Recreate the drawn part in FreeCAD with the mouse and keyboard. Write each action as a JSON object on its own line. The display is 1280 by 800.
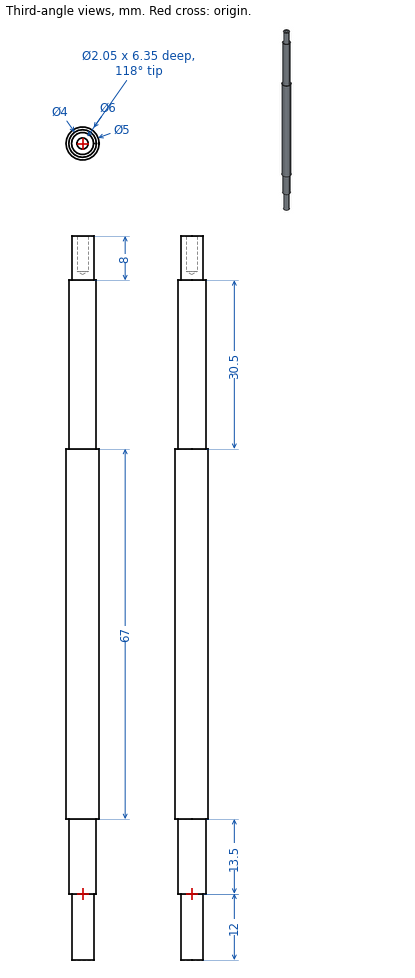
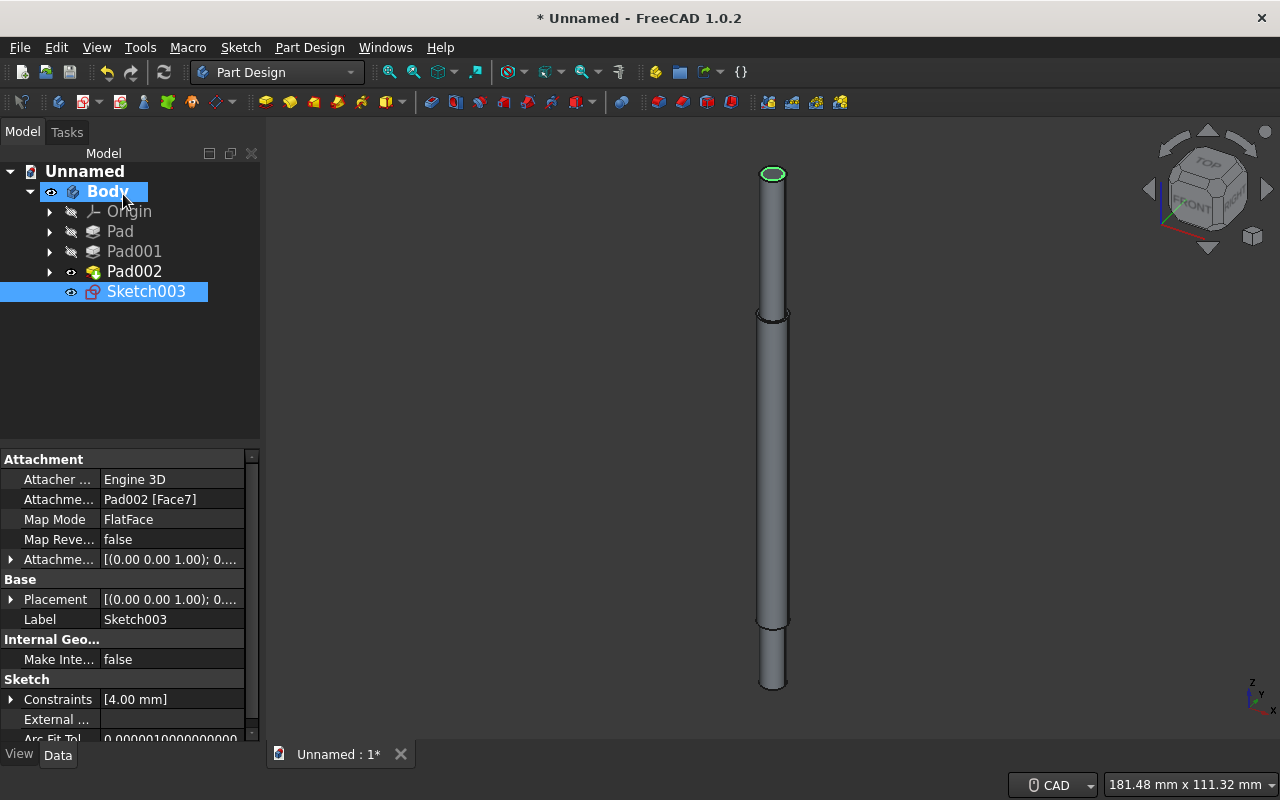
{"action": "left_click", "coordinate": [266, 102]}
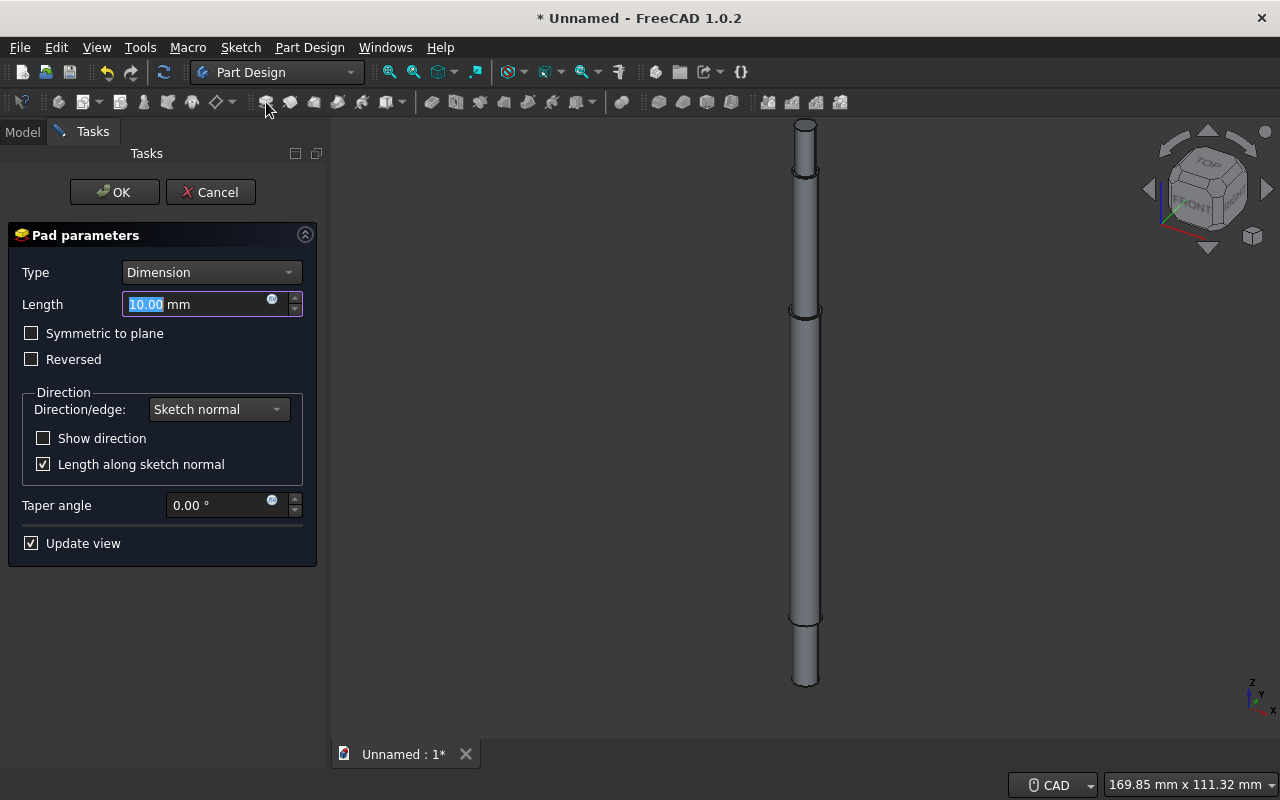
{"action": "type", "text": "8"}
{"action": "key", "text": "Tab"}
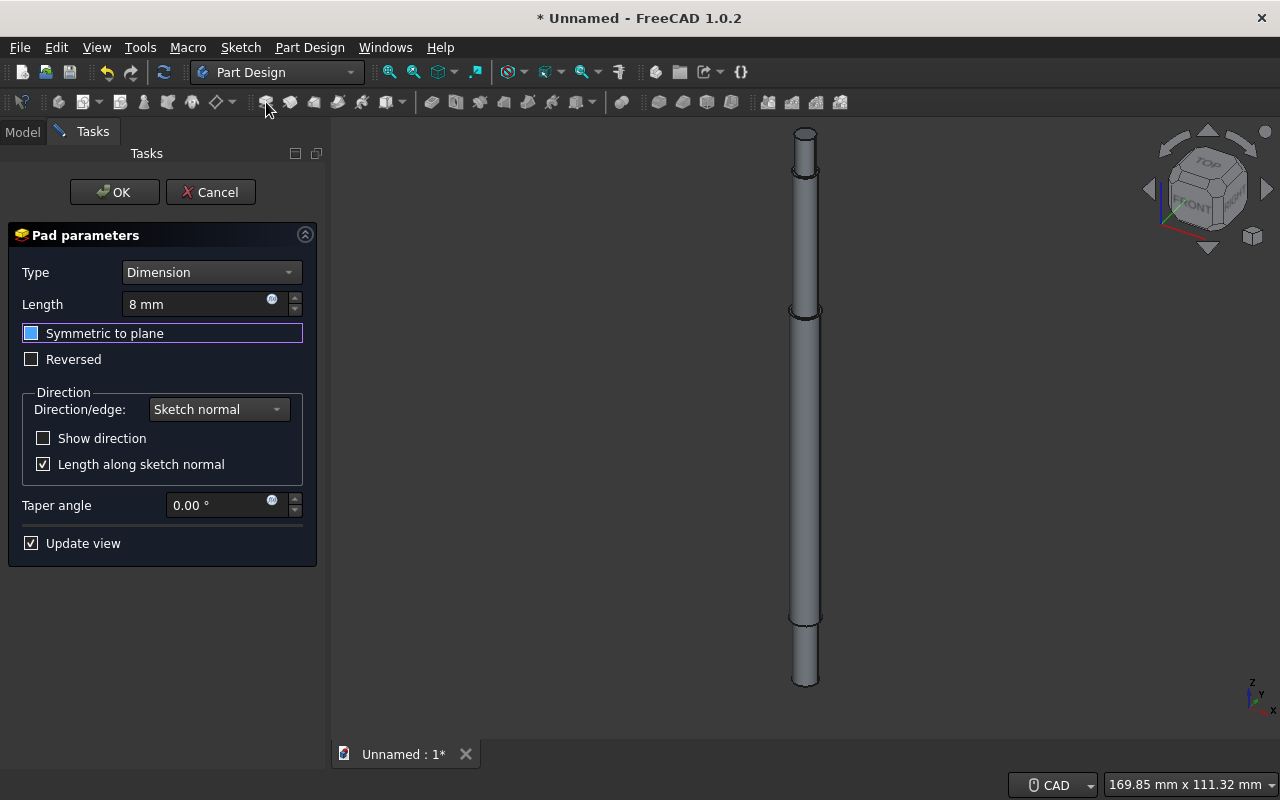
{"action": "left_click", "coordinate": [115, 192]}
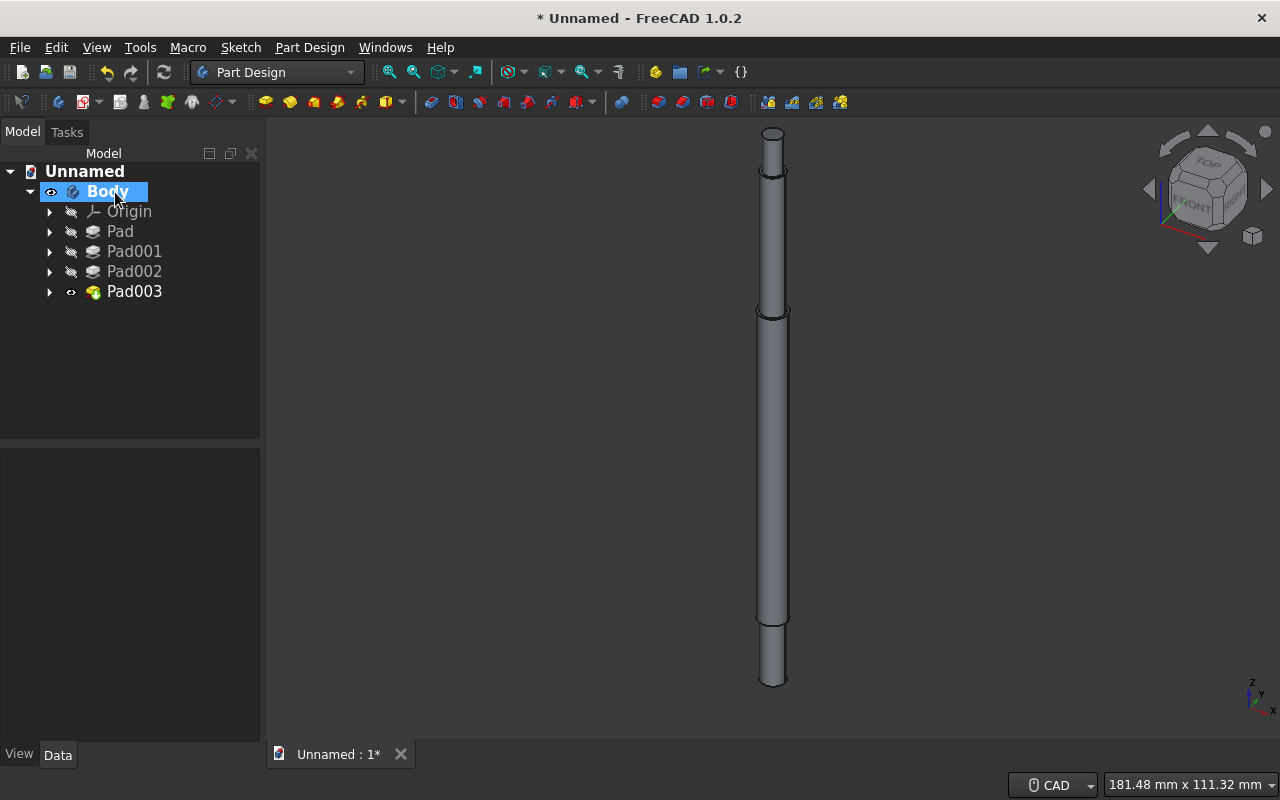
{"action": "left_click", "coordinate": [50, 212]}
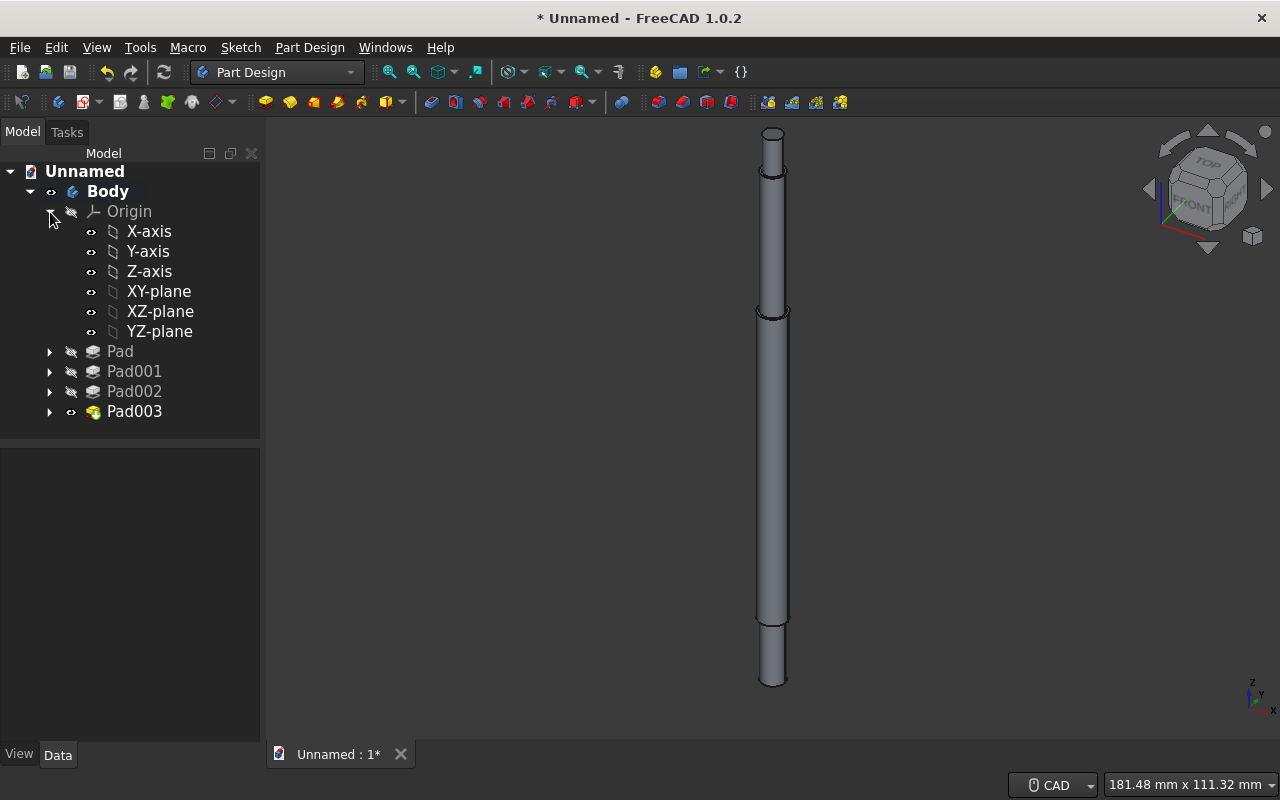
{"action": "left_click", "coordinate": [136, 292]}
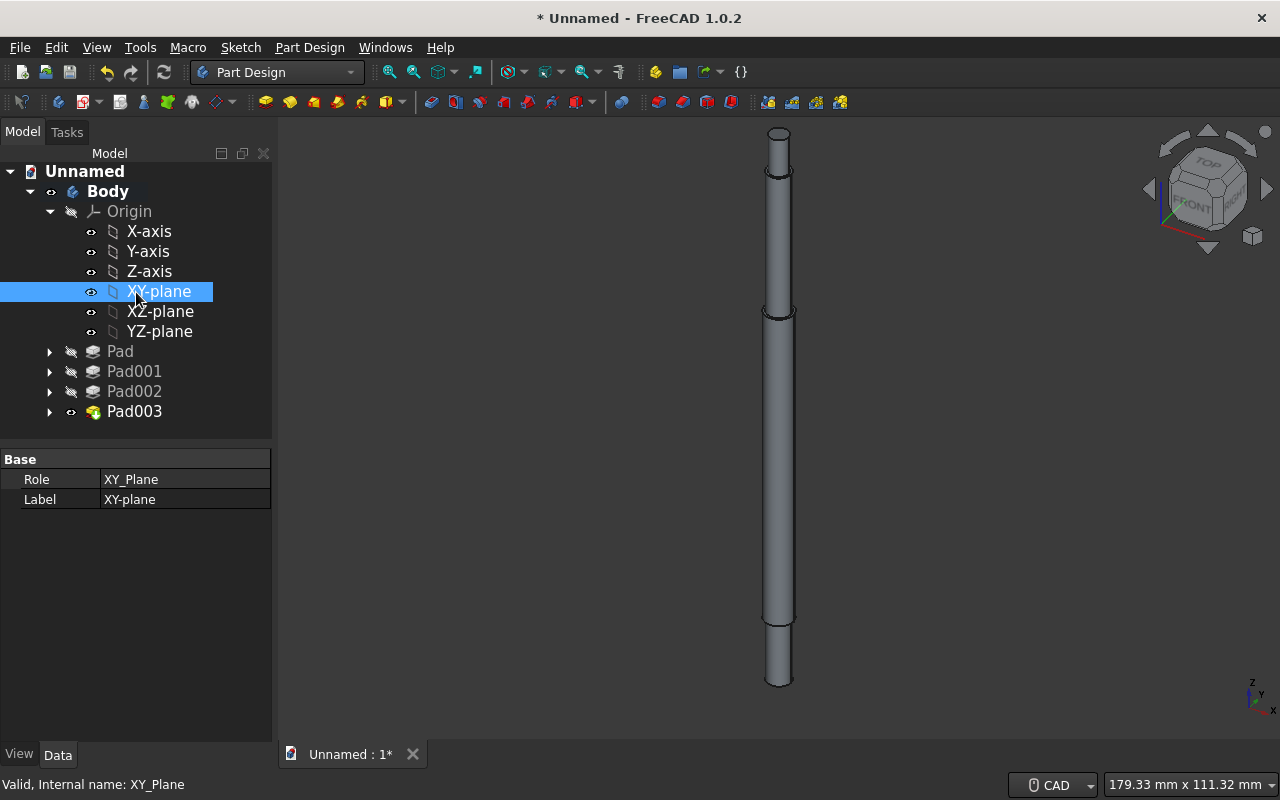
{"action": "left_click", "coordinate": [216, 102]}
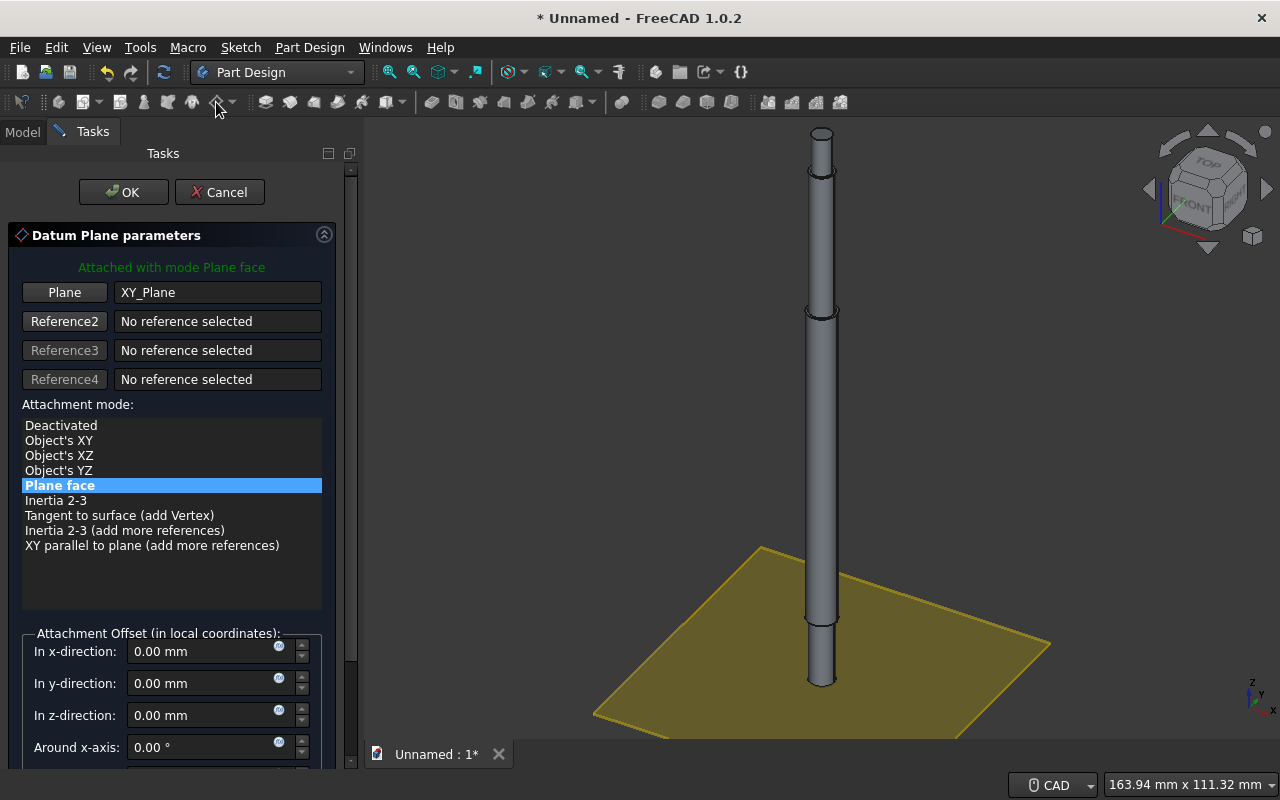
{"action": "triple_click", "coordinate": [210, 715]}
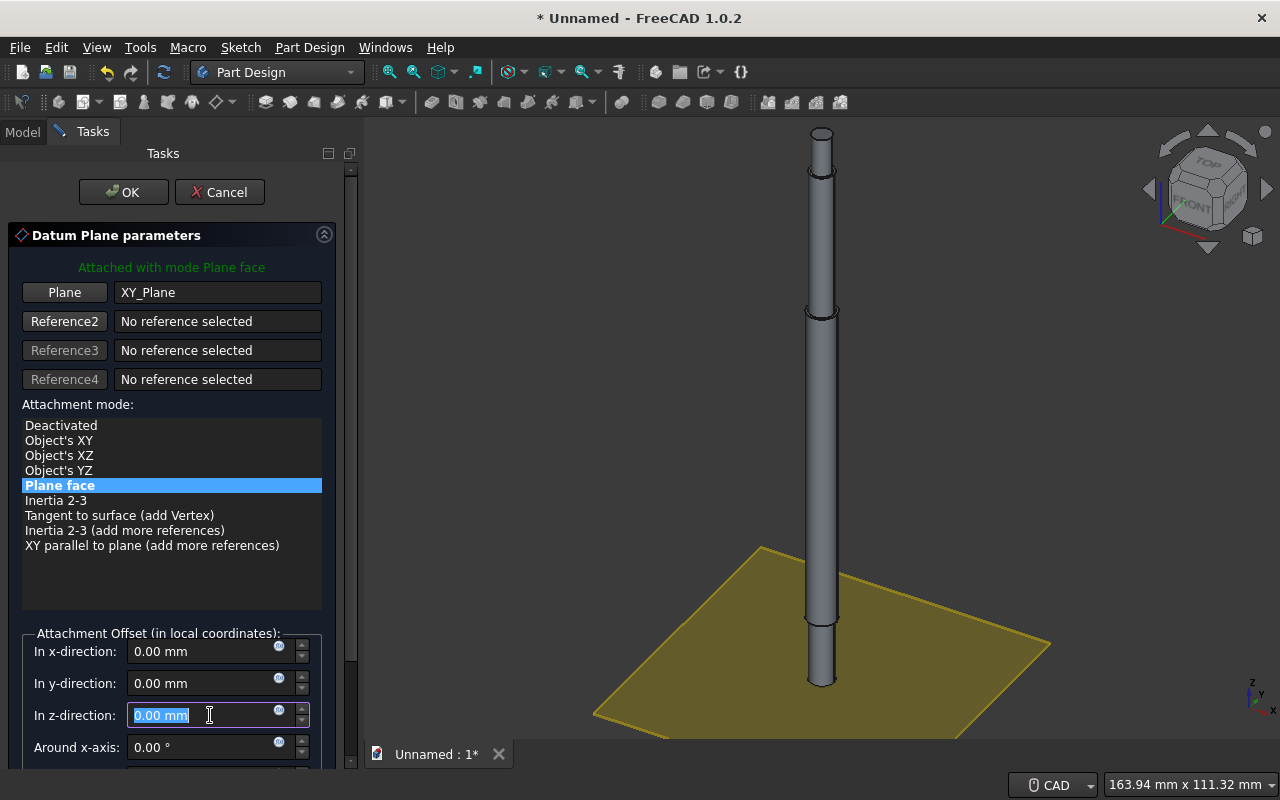
{"action": "type", "text": "-12"}
{"action": "key", "text": "Tab"}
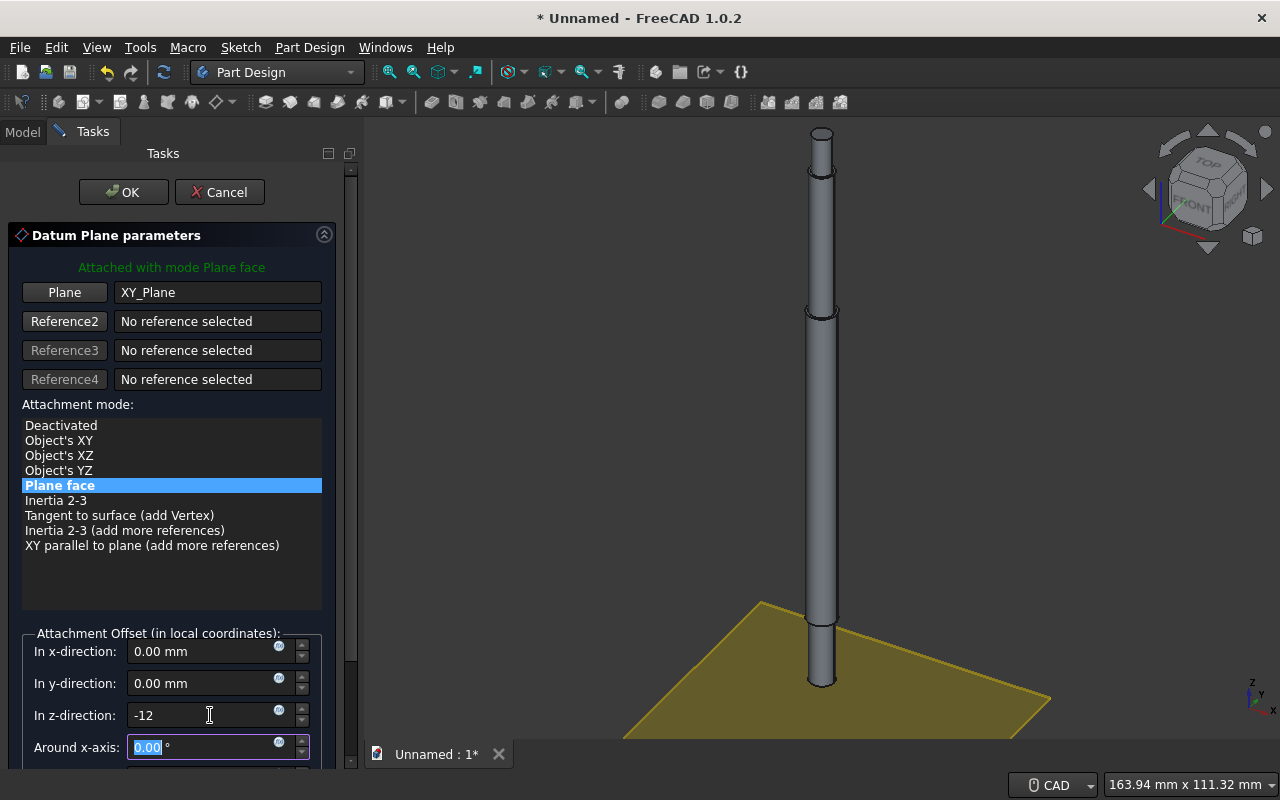
{"action": "left_click", "coordinate": [124, 192]}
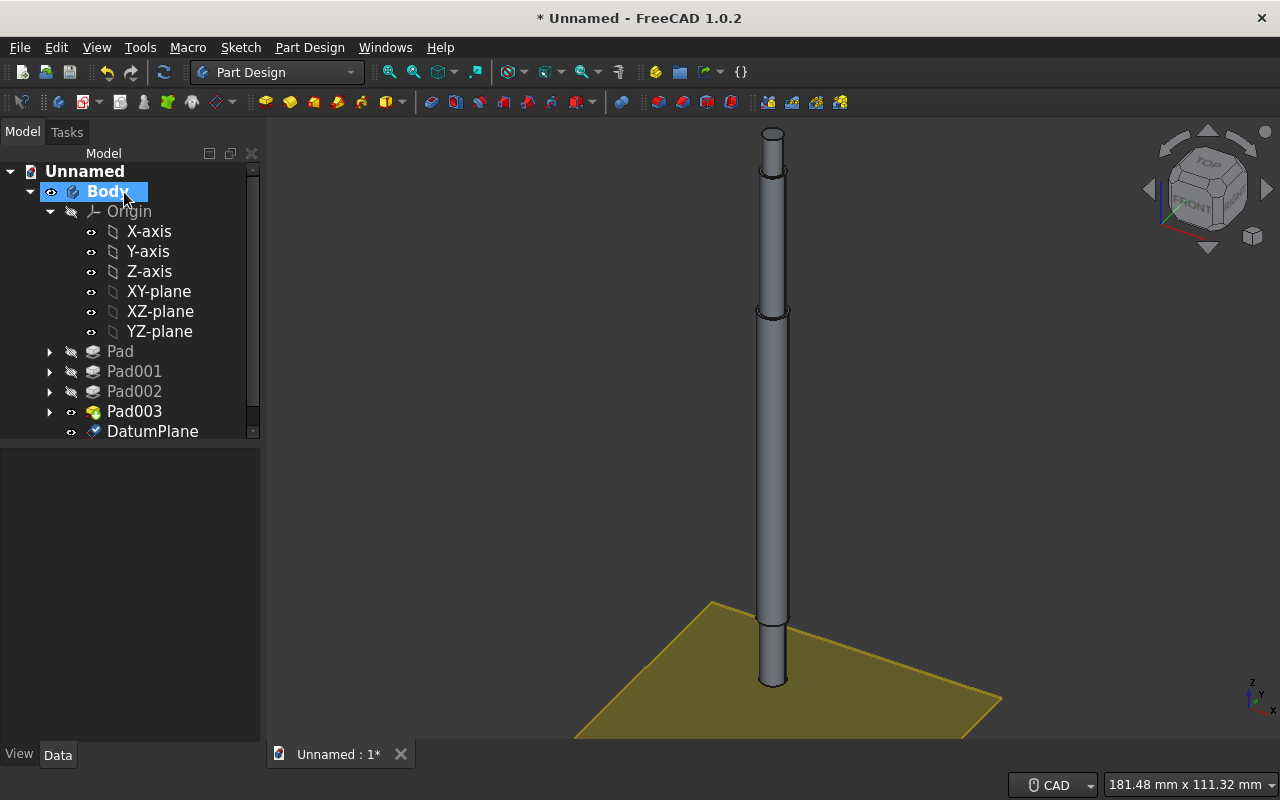
{"action": "left_click", "coordinate": [116, 432]}